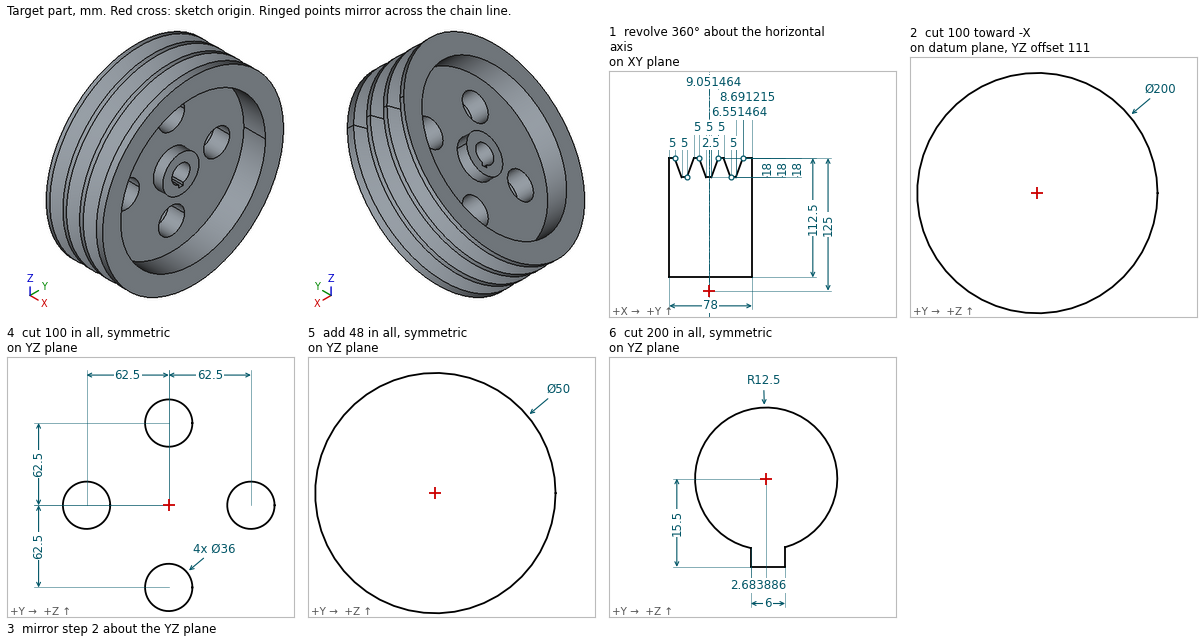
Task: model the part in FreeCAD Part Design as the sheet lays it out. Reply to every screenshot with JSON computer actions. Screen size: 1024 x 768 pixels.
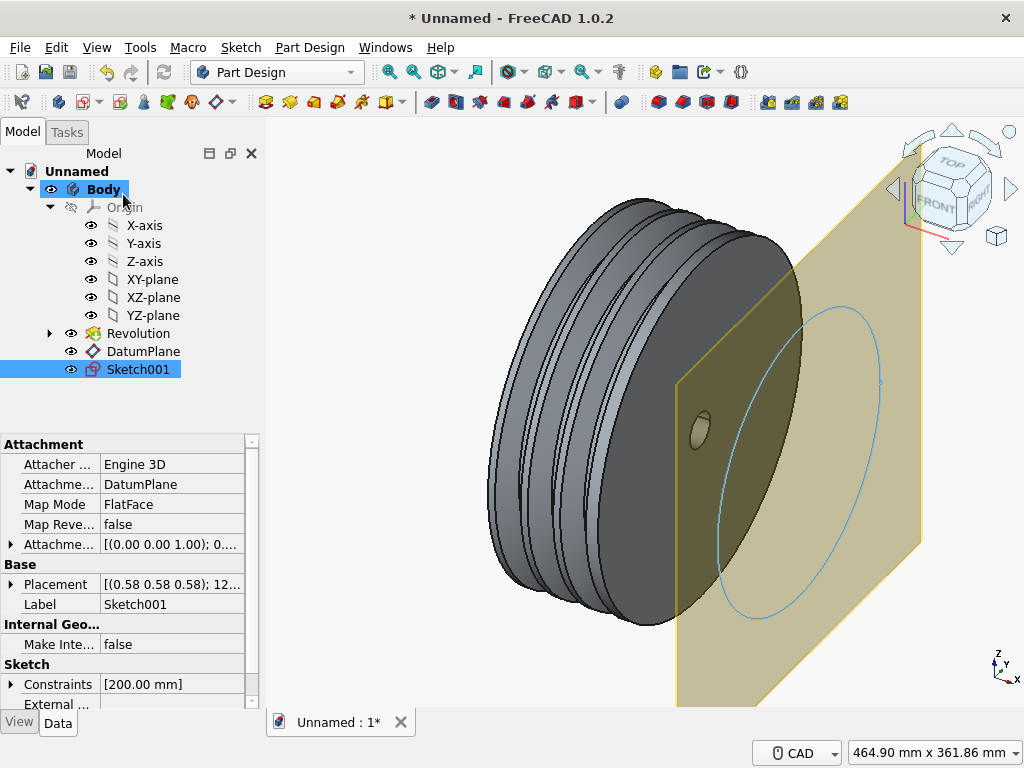
{"action": "left_click", "coordinate": [432, 102]}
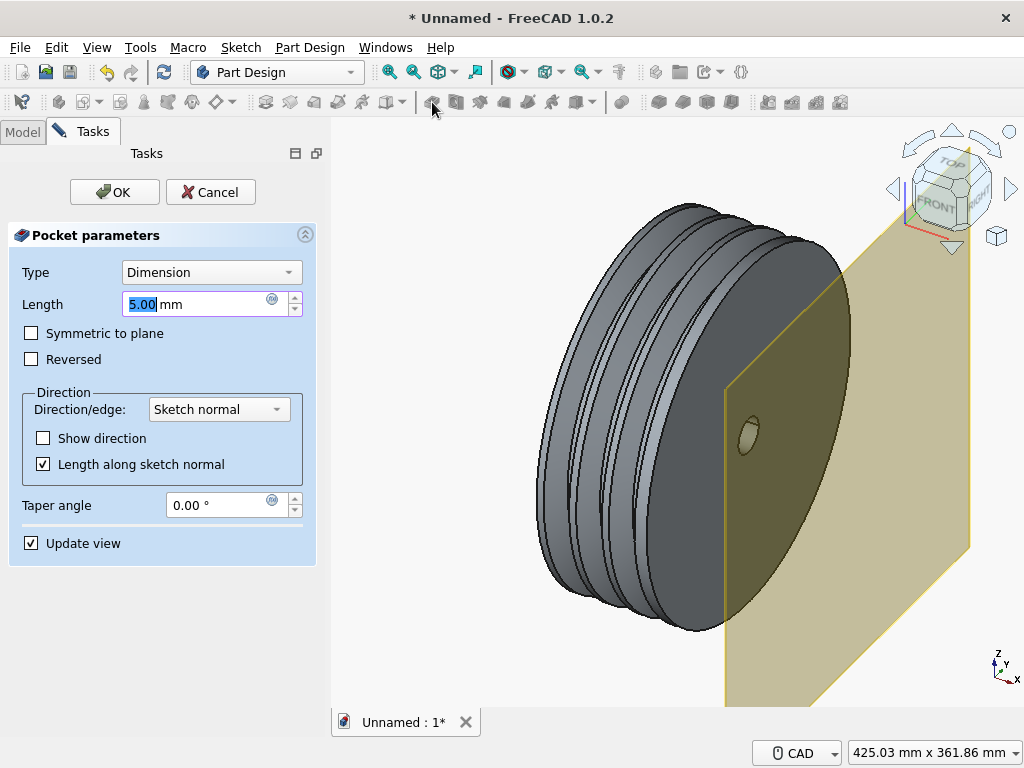
{"action": "type", "text": "100"}
{"action": "key", "text": "Tab"}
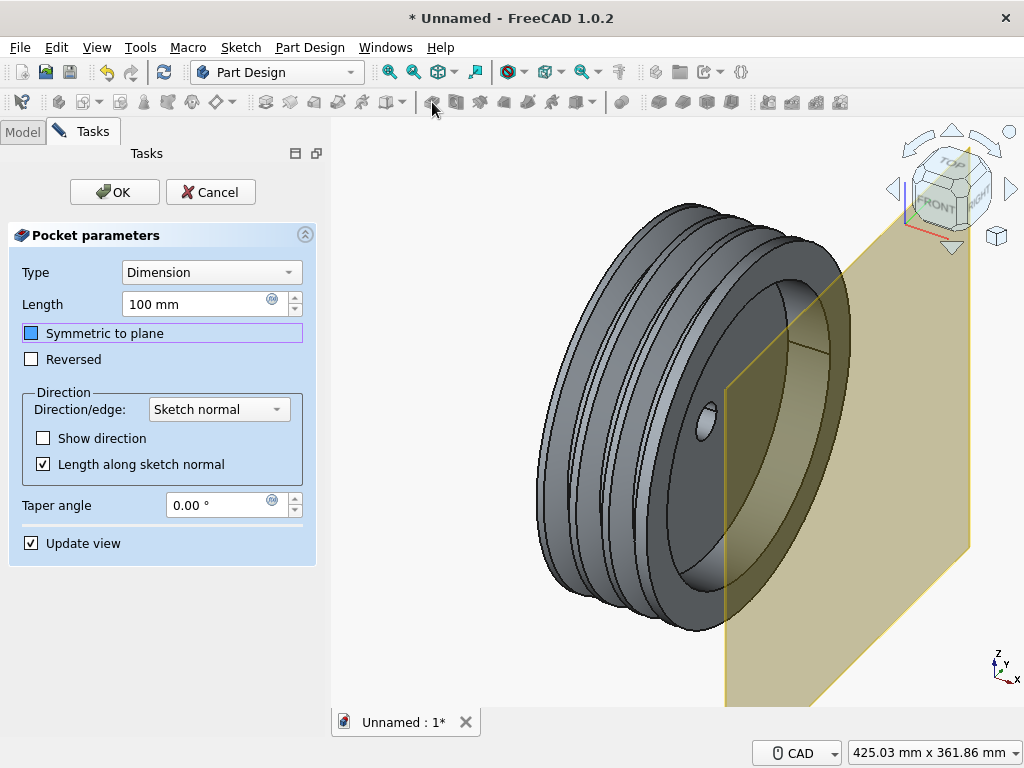
{"action": "left_click", "coordinate": [115, 192]}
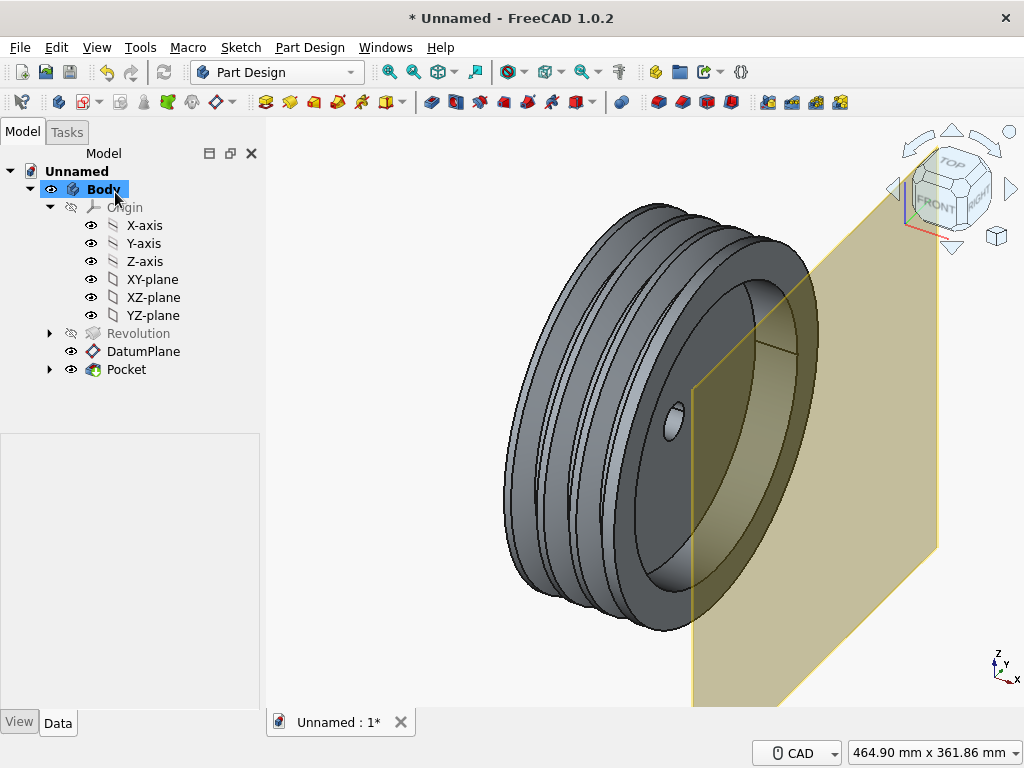
{"action": "left_click", "coordinate": [116, 351]}
{"action": "key", "text": "space"}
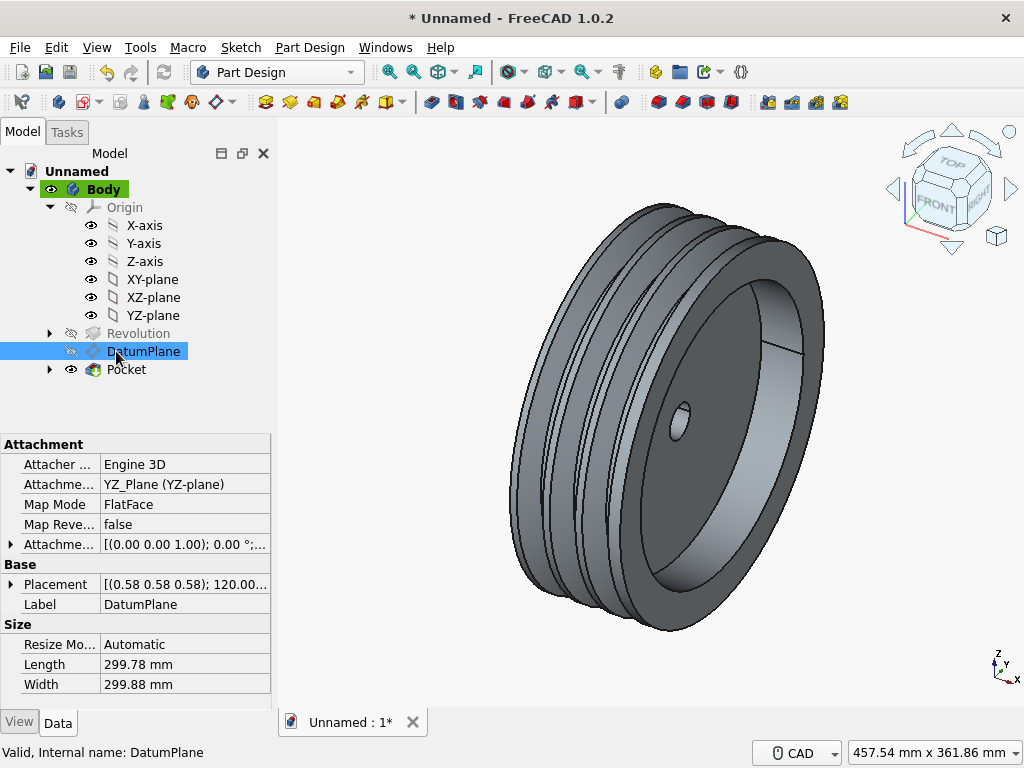
{"action": "left_click", "coordinate": [116, 369]}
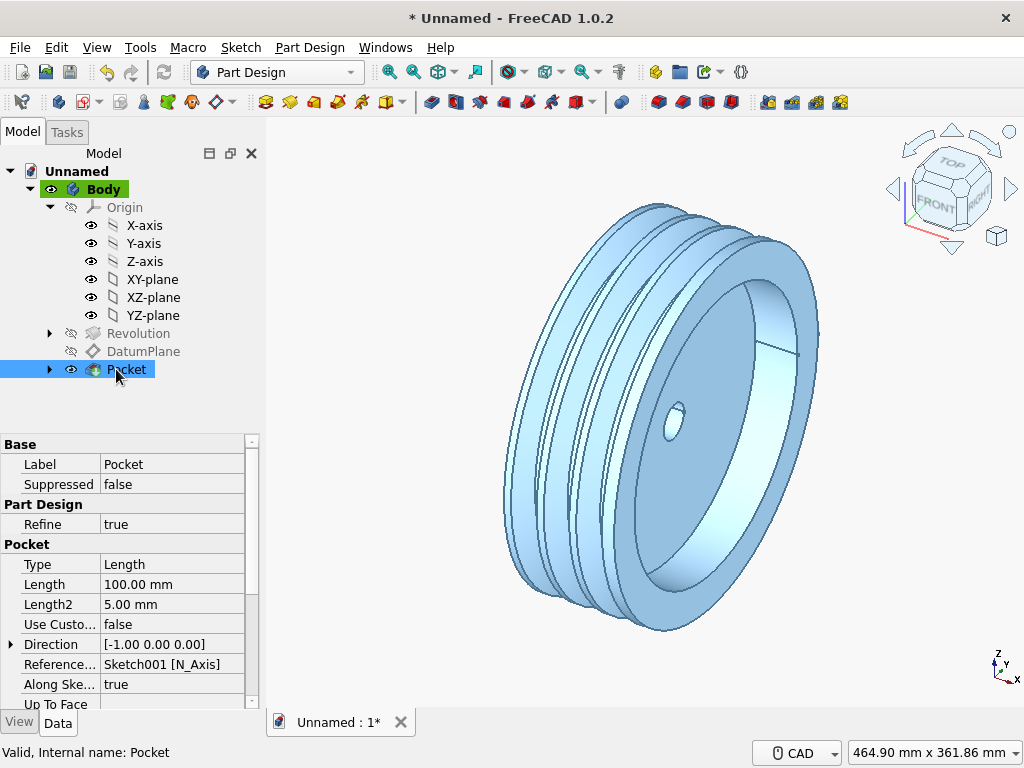
{"action": "left_click", "coordinate": [768, 102]}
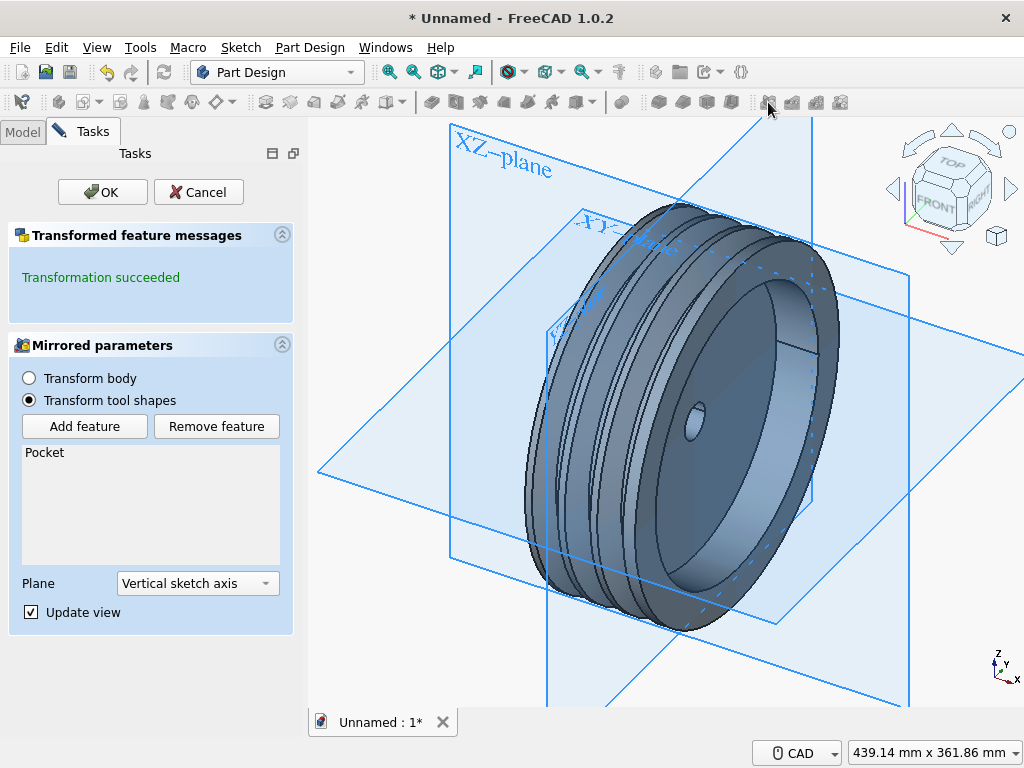
{"action": "left_click", "coordinate": [198, 584]}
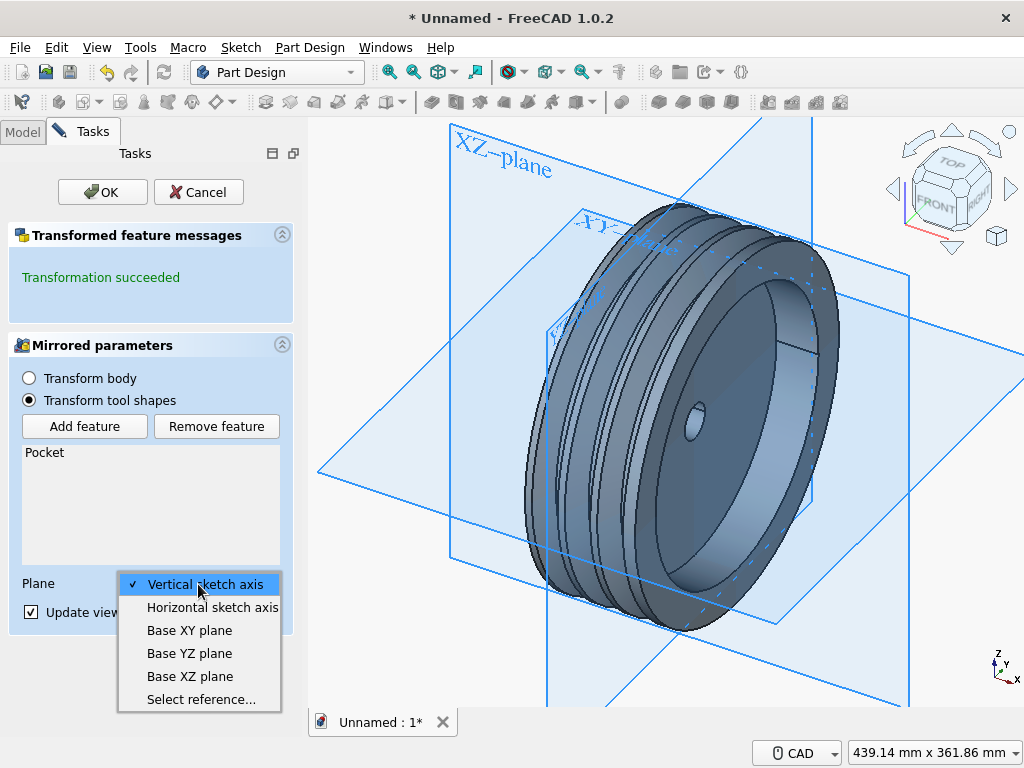
{"action": "left_click", "coordinate": [198, 654]}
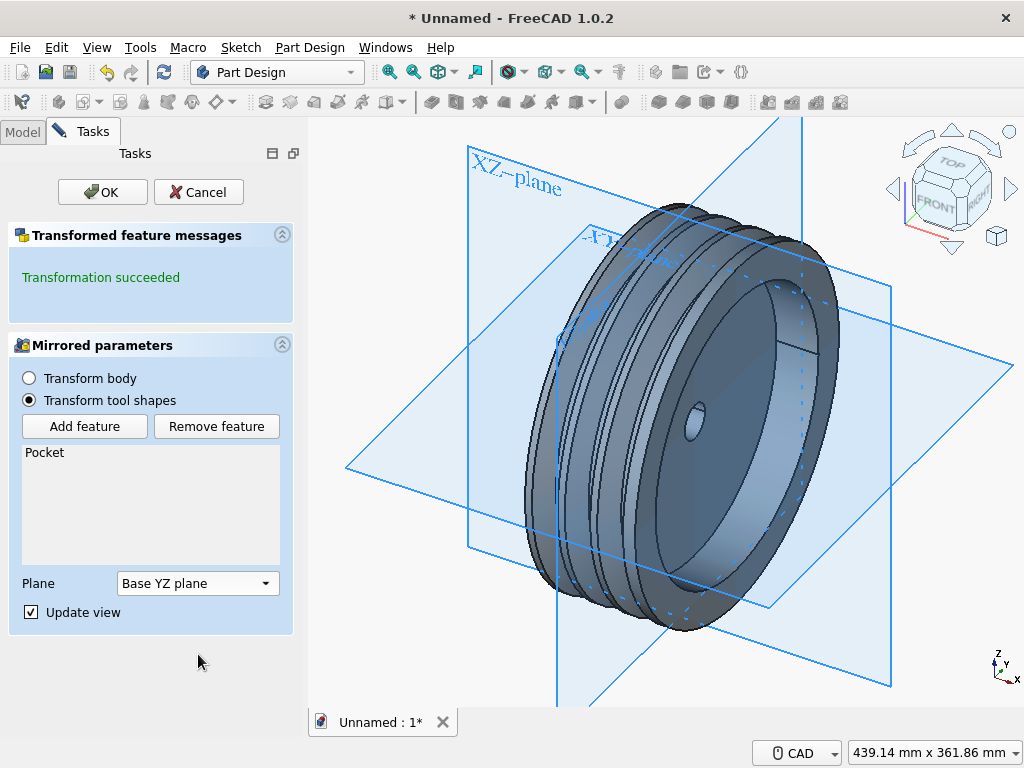
{"action": "left_click", "coordinate": [103, 192]}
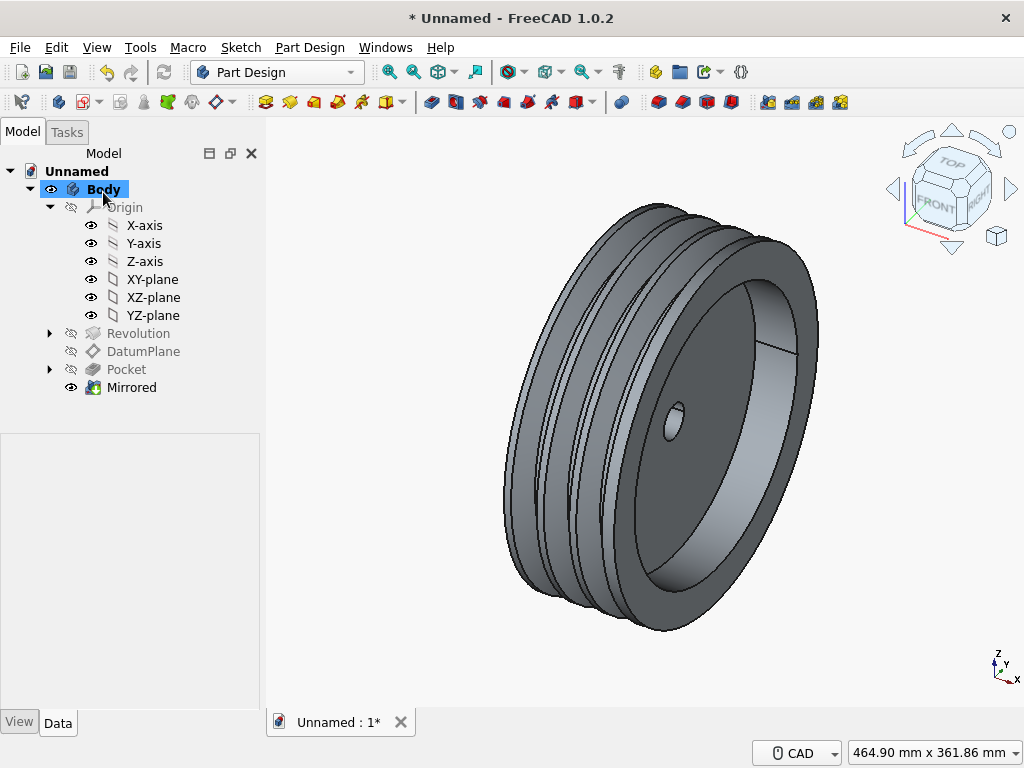
{"action": "left_click", "coordinate": [84, 102]}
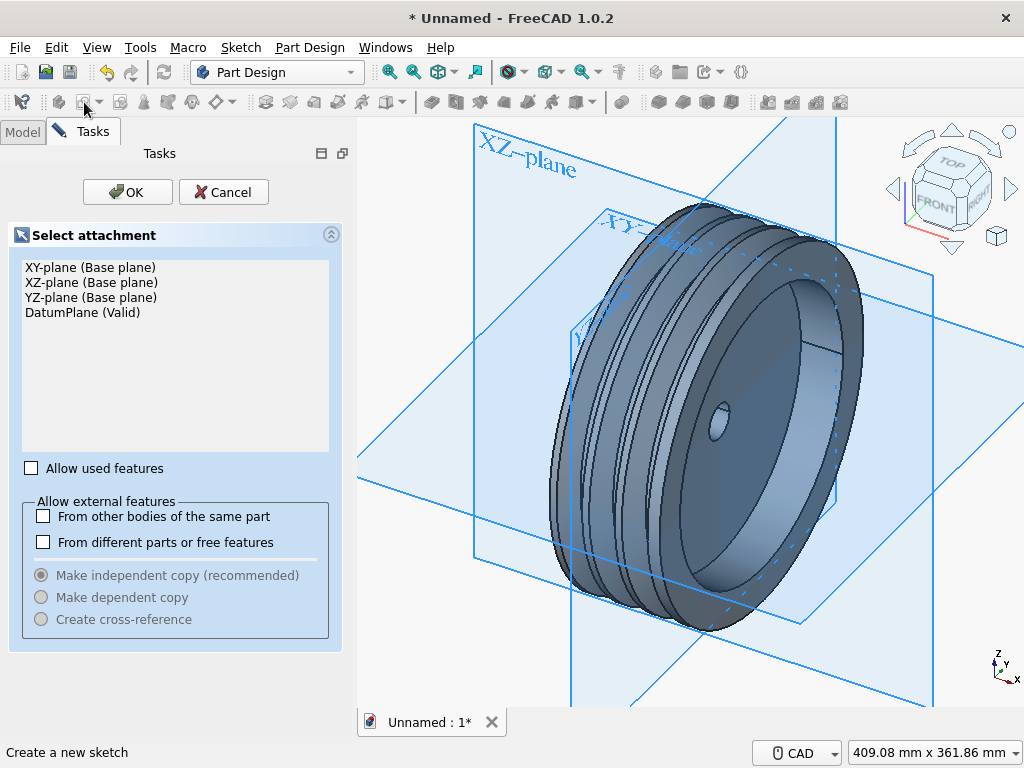
{"action": "left_click", "coordinate": [82, 298]}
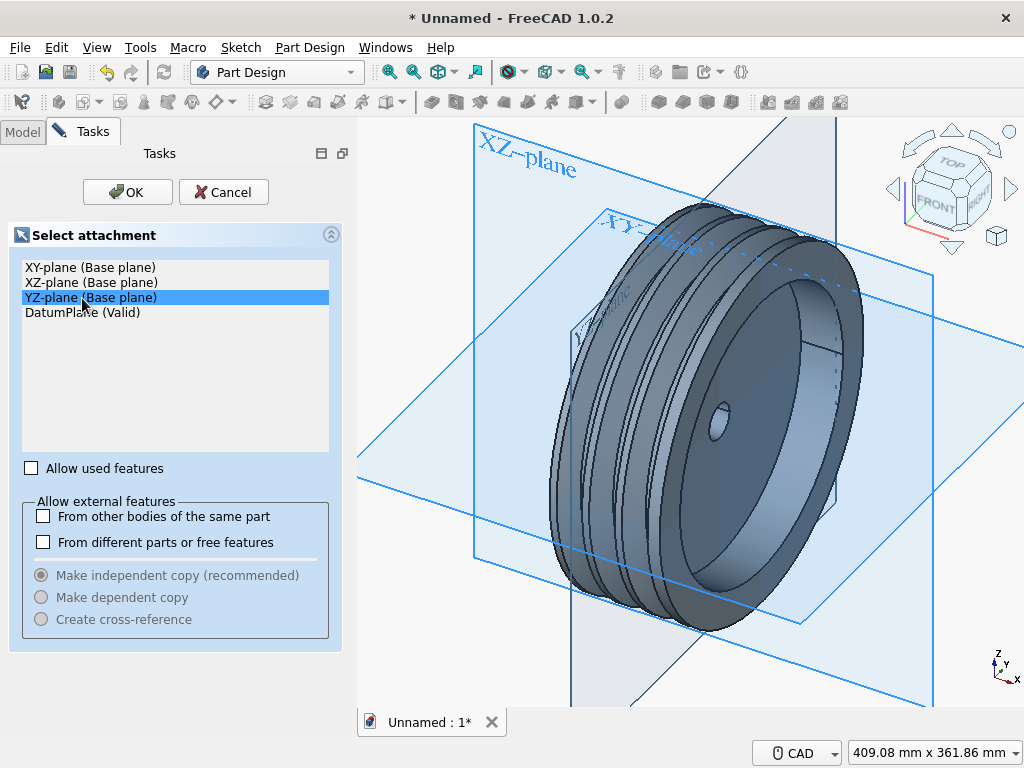
{"action": "left_click", "coordinate": [128, 192]}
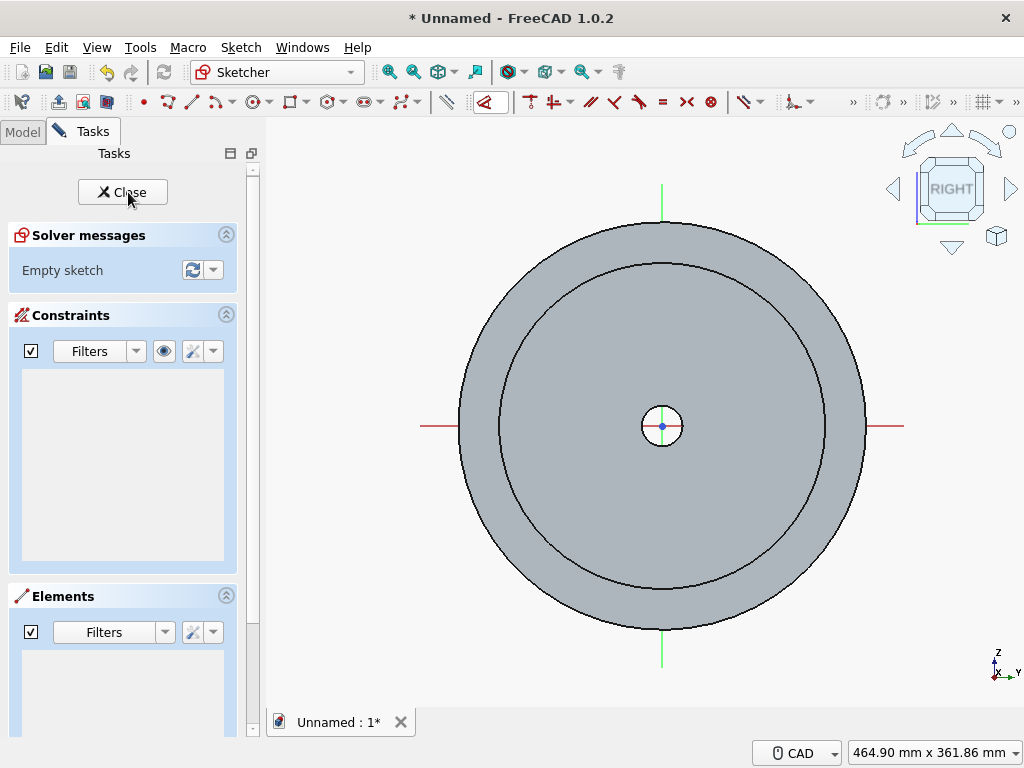
{"action": "left_click", "coordinate": [108, 102]}